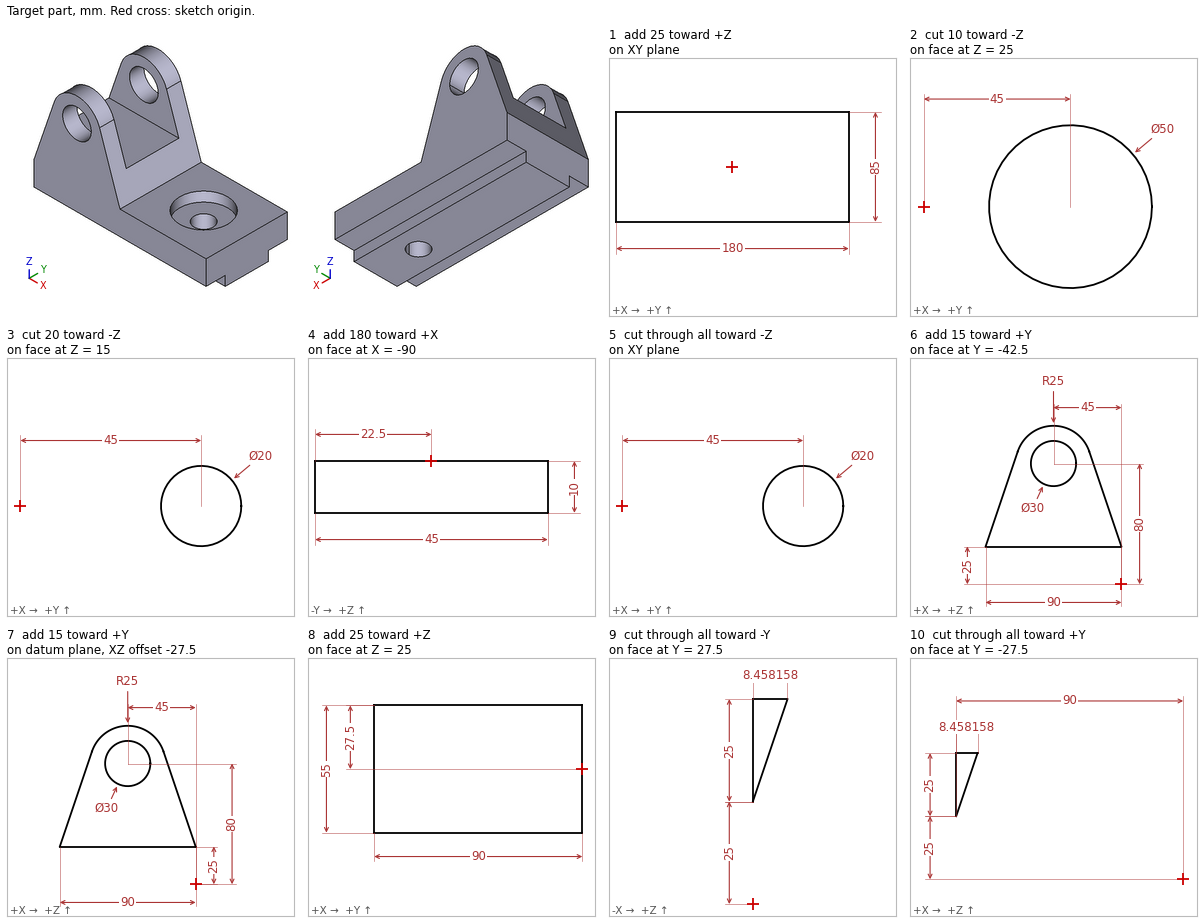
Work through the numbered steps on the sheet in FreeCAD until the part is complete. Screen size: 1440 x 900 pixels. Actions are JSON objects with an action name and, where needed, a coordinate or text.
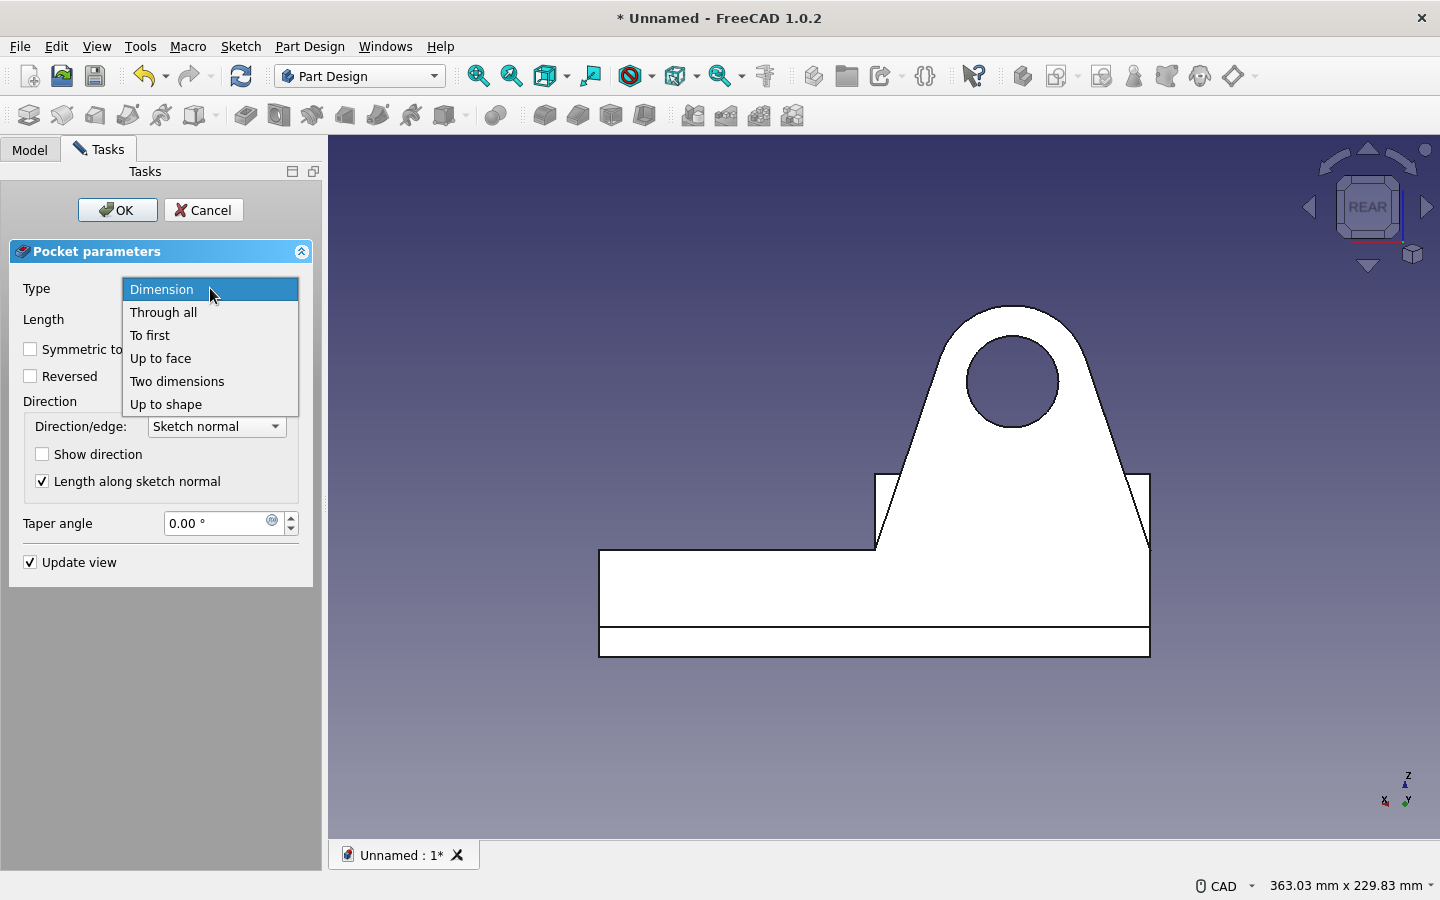
{"action": "left_click", "coordinate": [208, 312]}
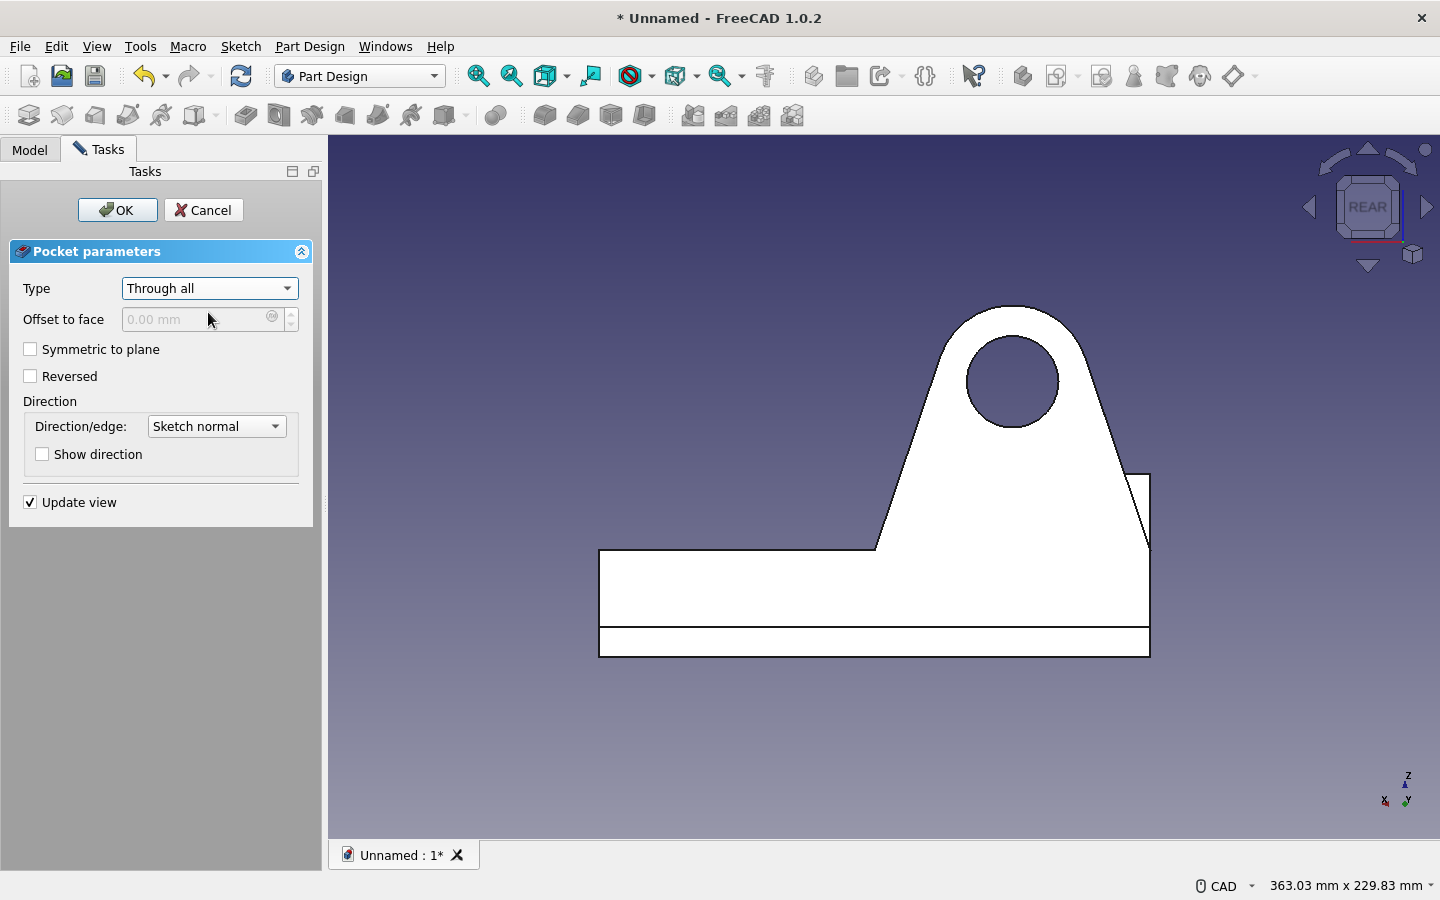
{"action": "left_click", "coordinate": [118, 210]}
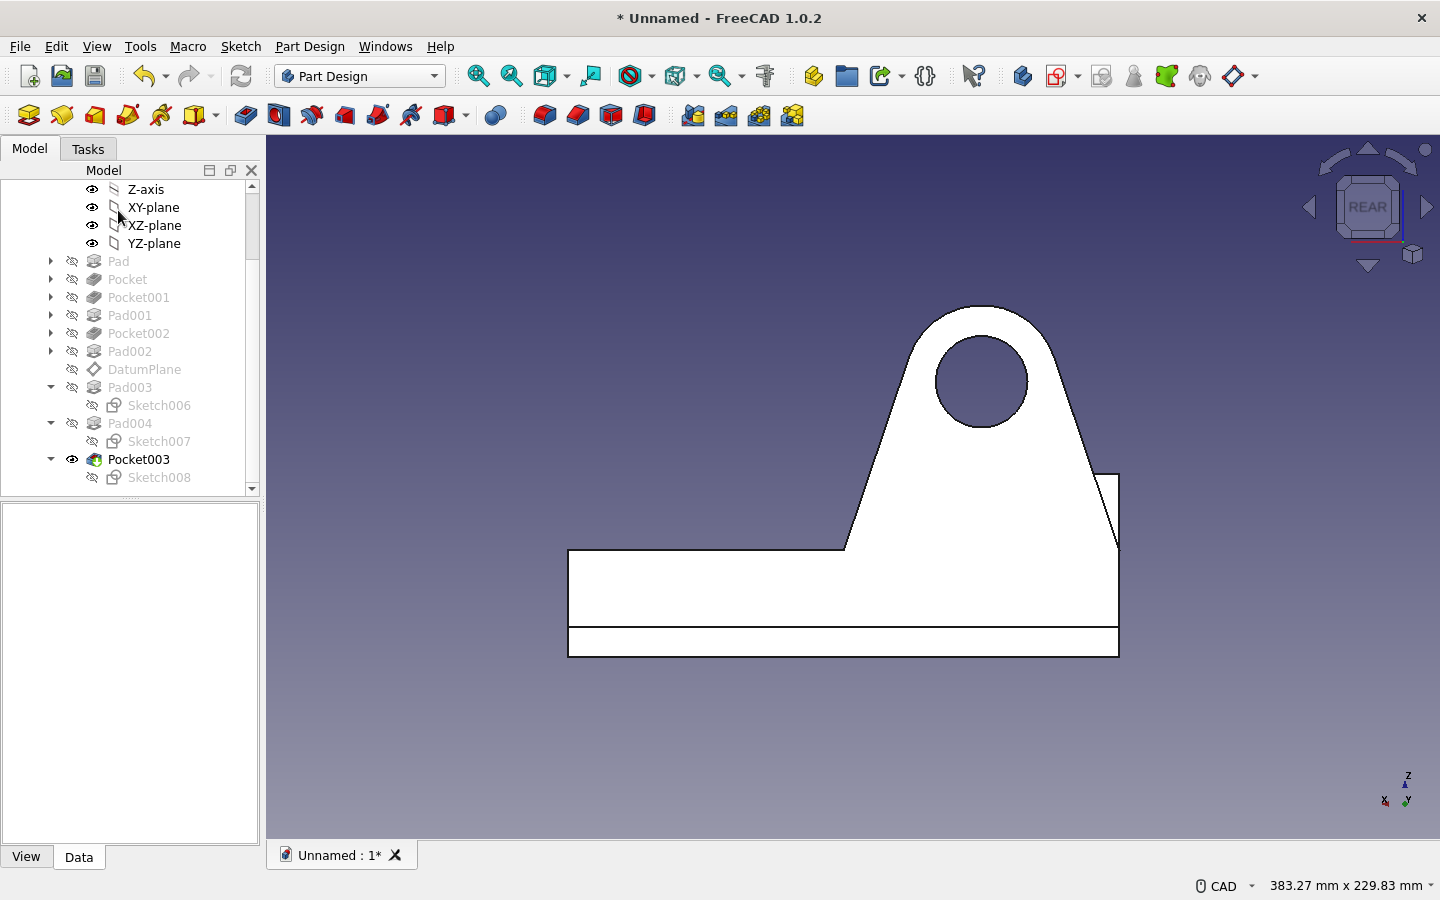
{"action": "key", "text": "0"}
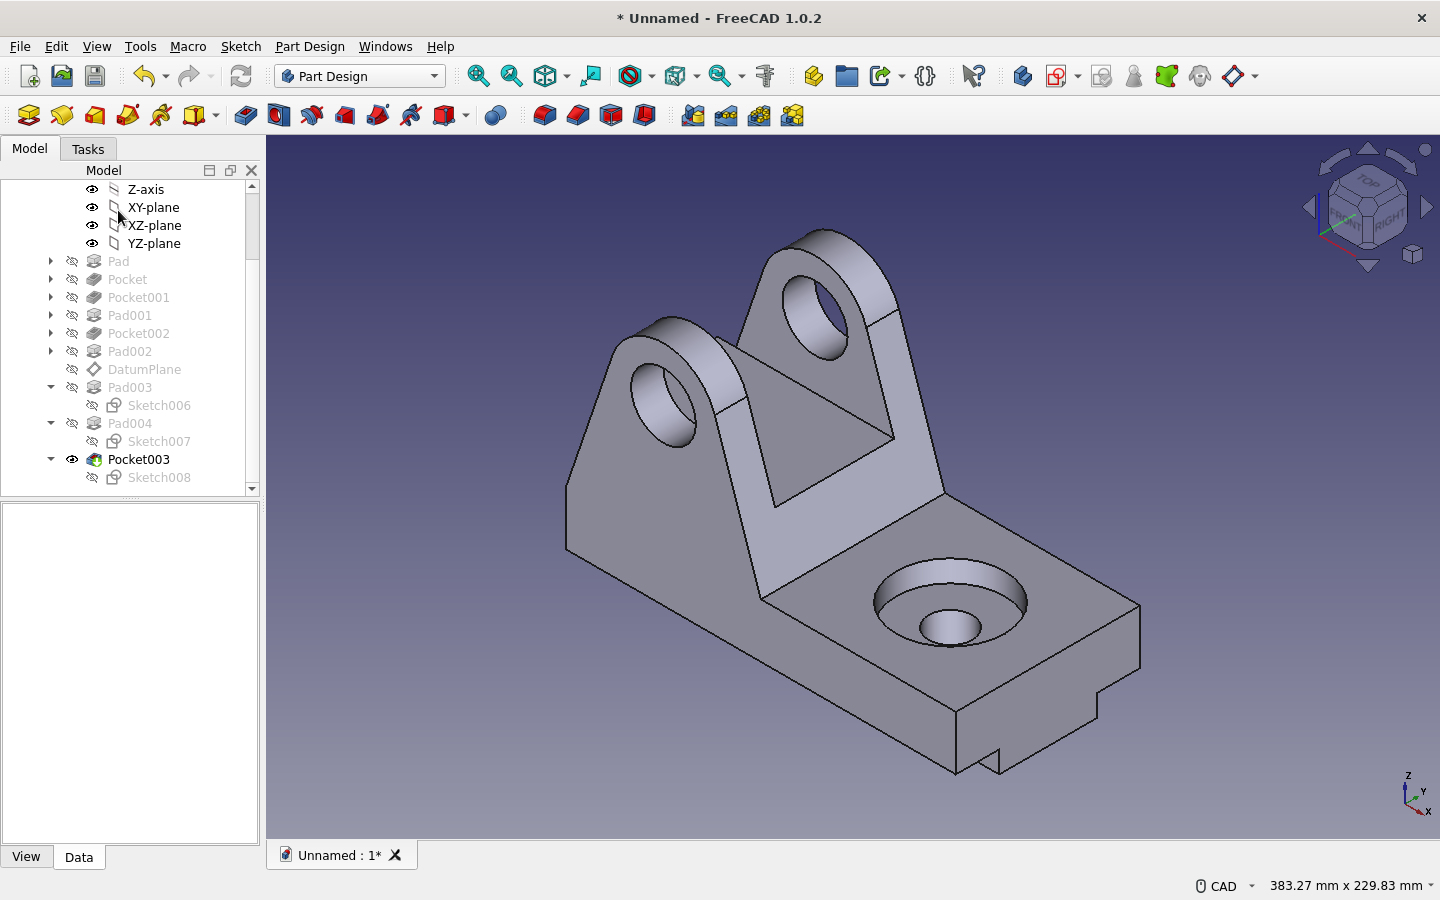
{"action": "key", "text": "1"}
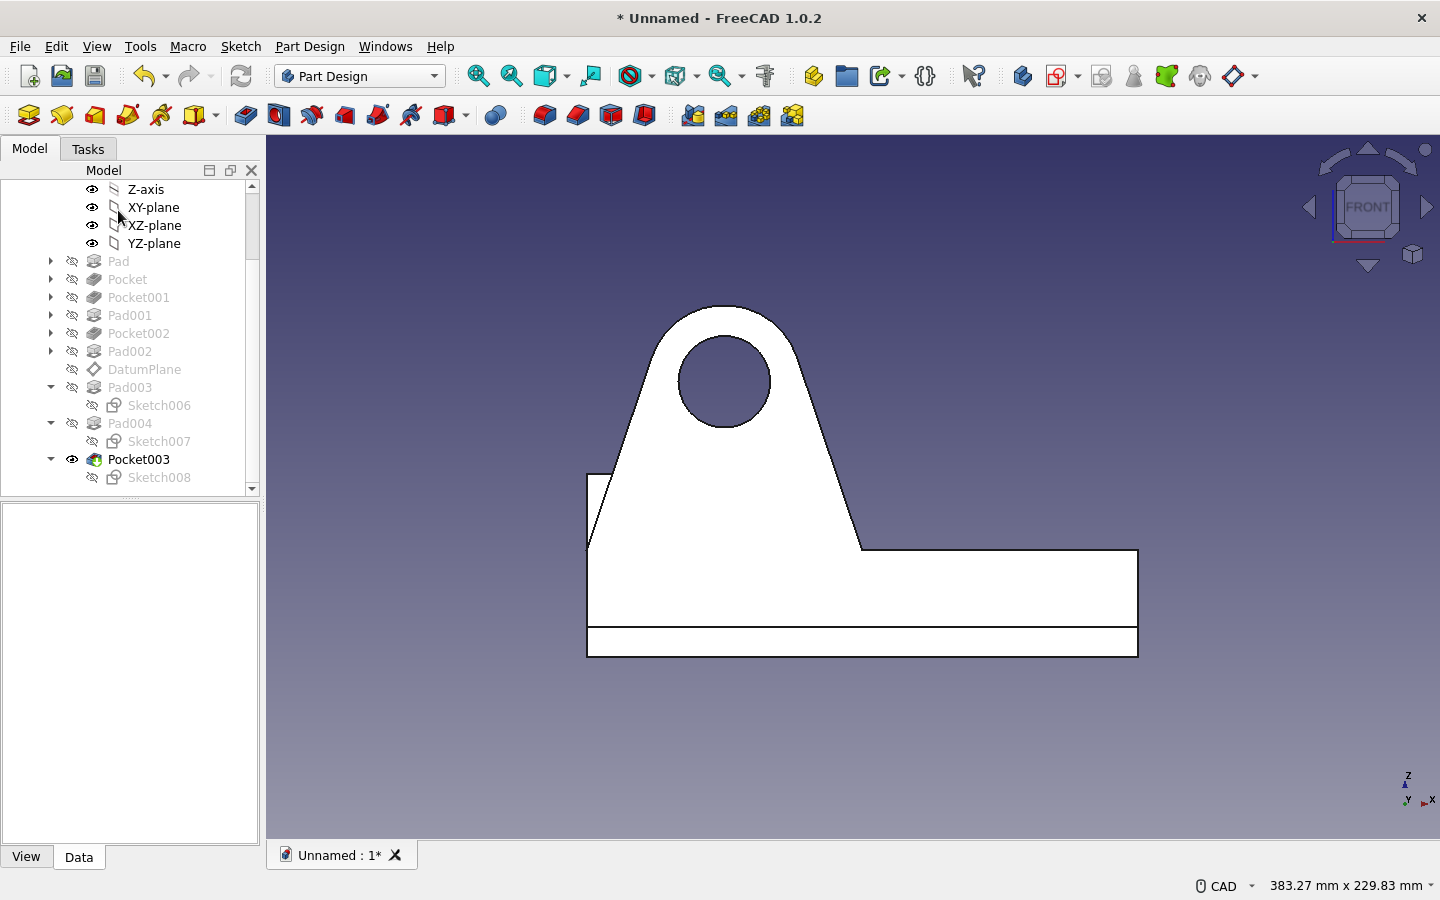
{"action": "left_click", "coordinate": [596, 489]}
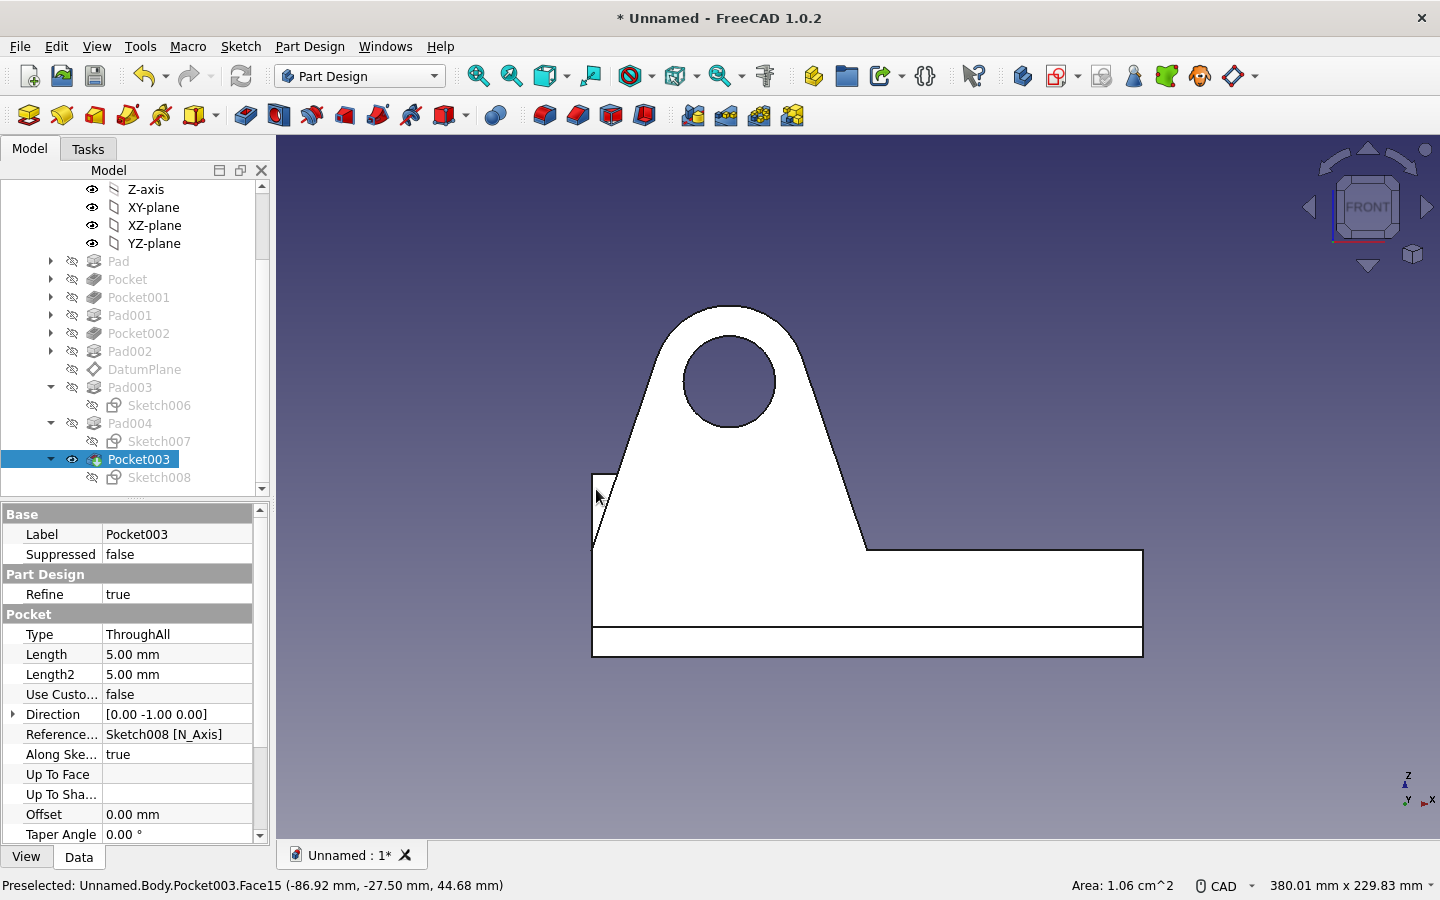
{"action": "left_click", "coordinate": [1056, 76]}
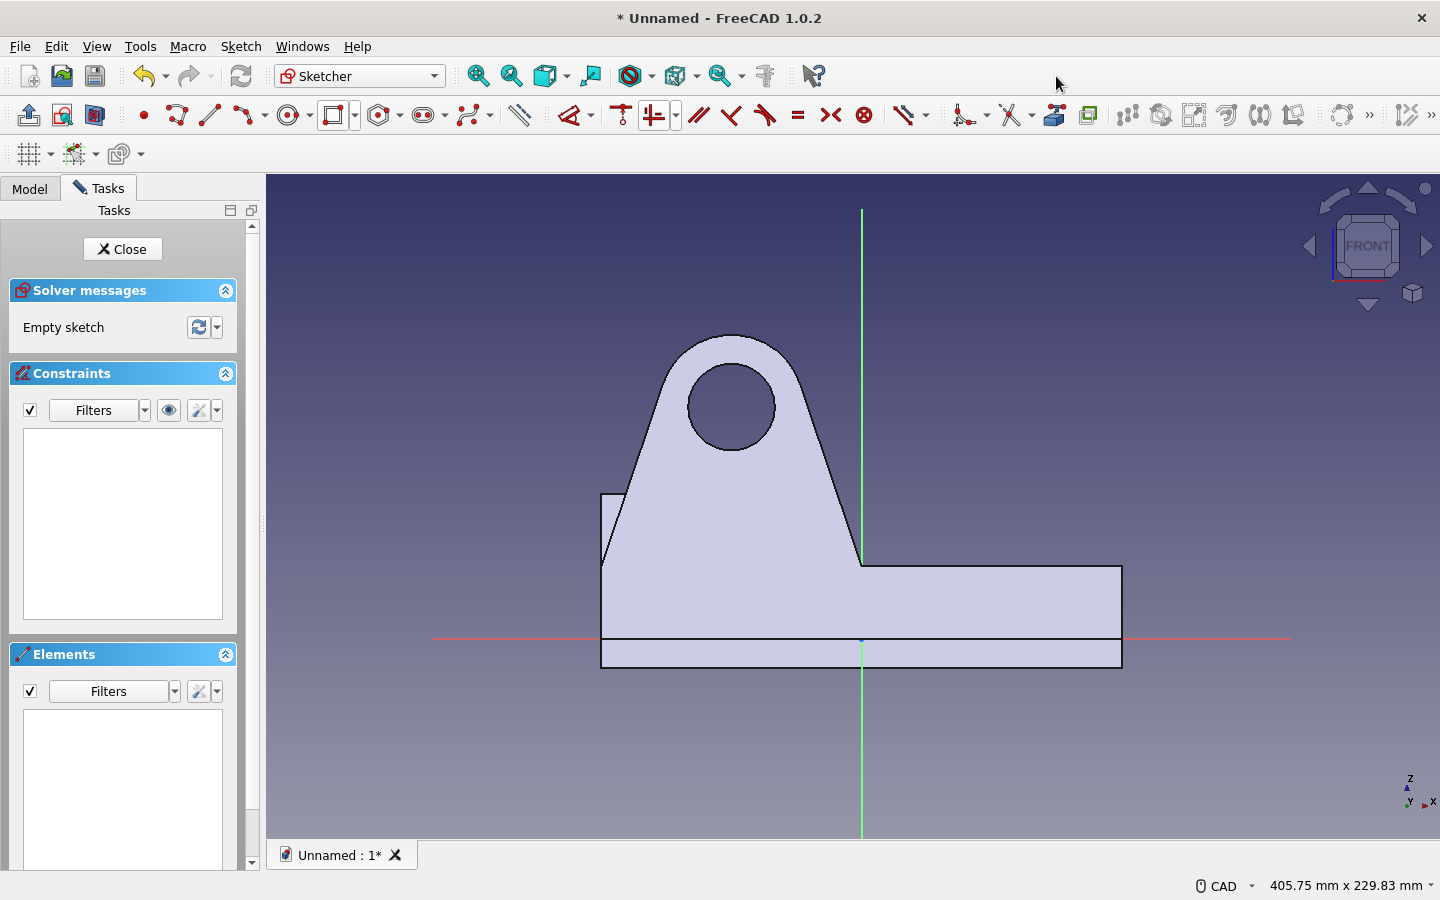
{"action": "left_click", "coordinate": [95, 116]}